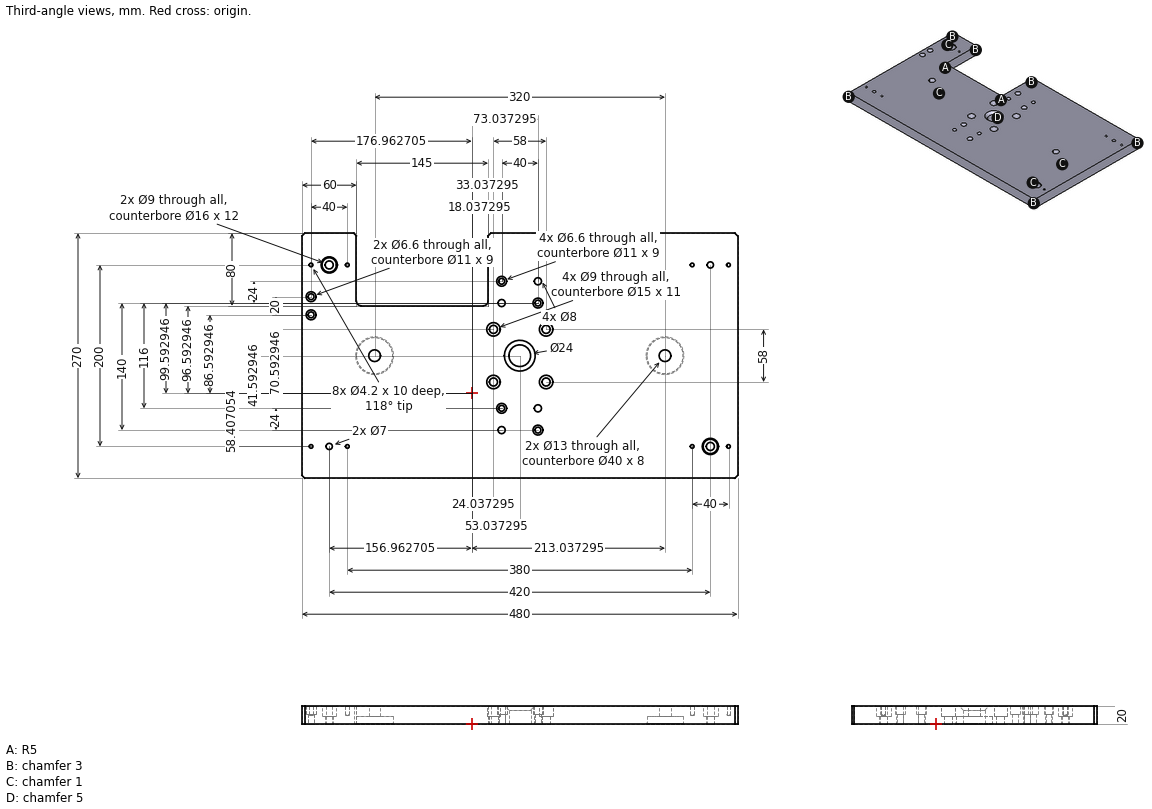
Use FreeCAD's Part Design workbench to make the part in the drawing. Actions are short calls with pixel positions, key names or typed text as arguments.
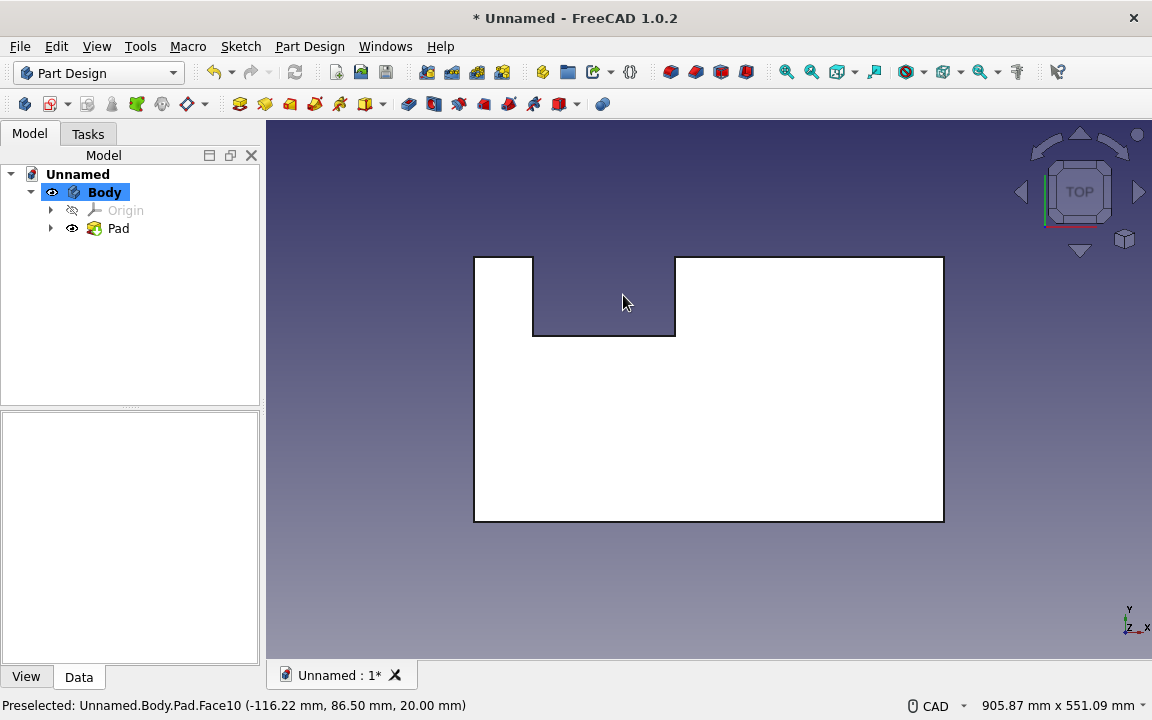
scroll(533, 335, up, 4)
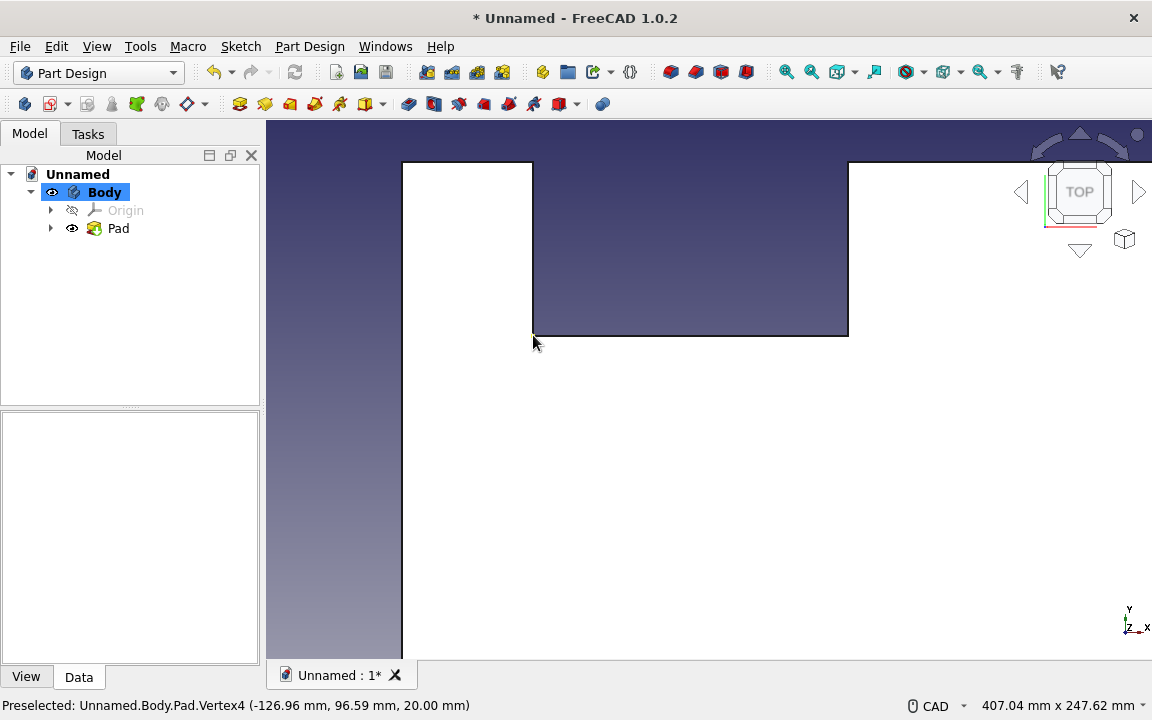
key(v)
key(f)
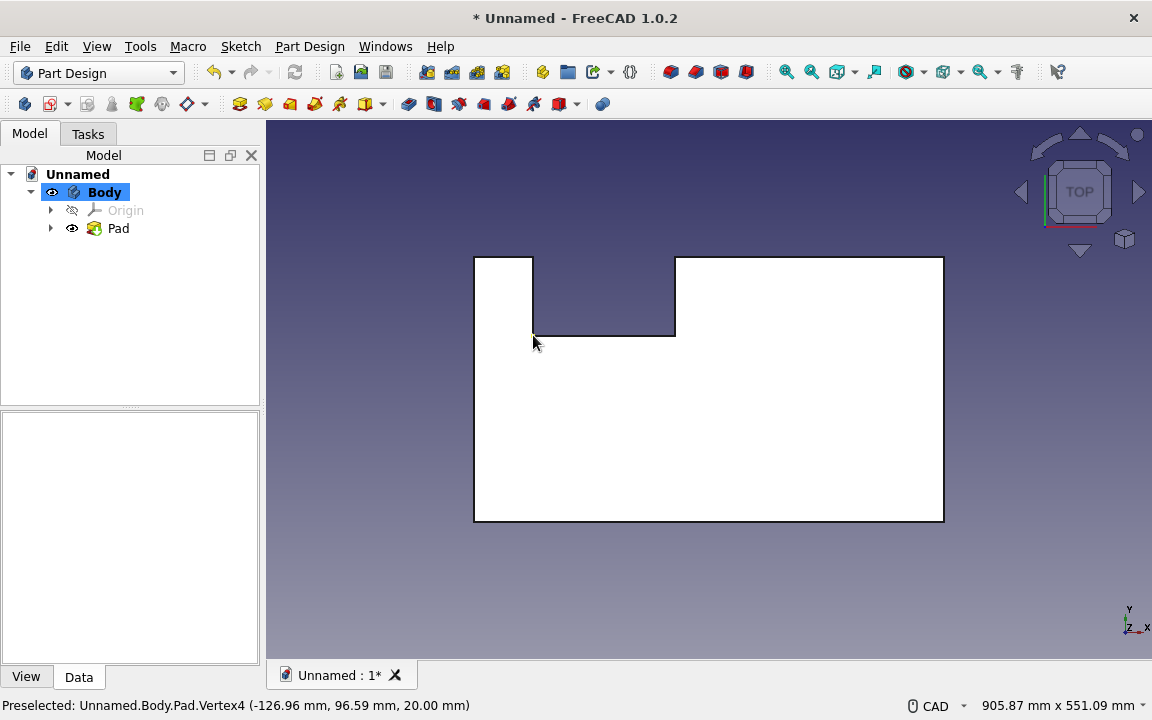
key(1)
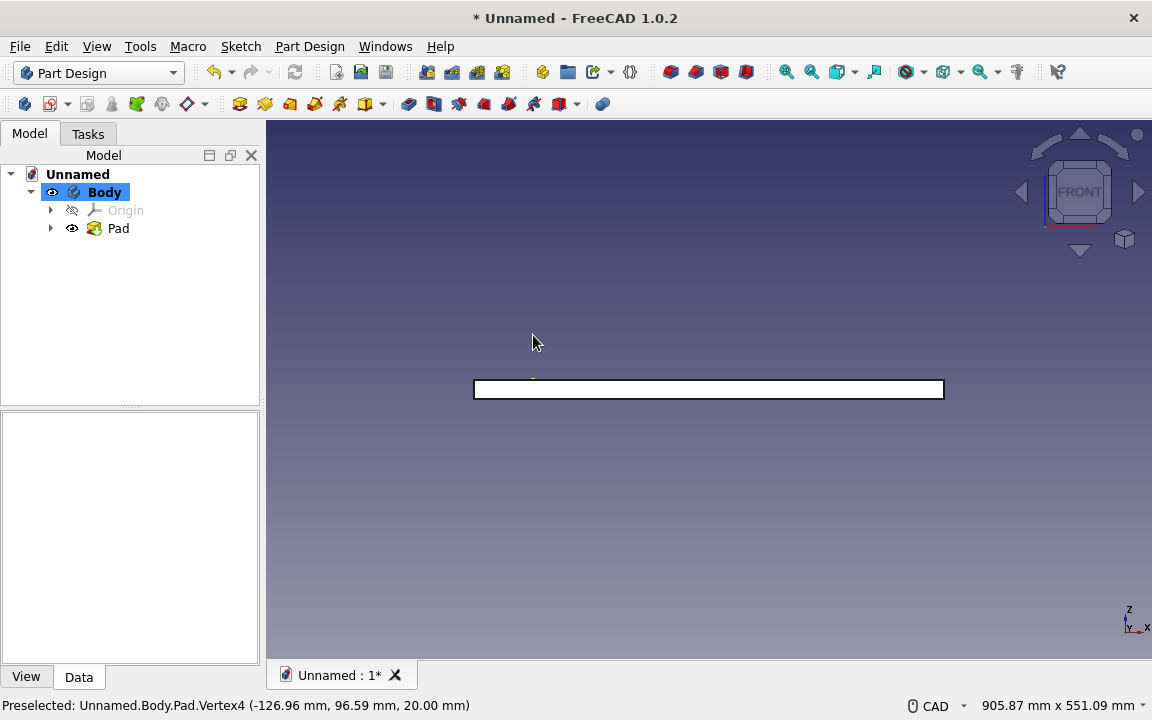
scroll(533, 388, up, 4)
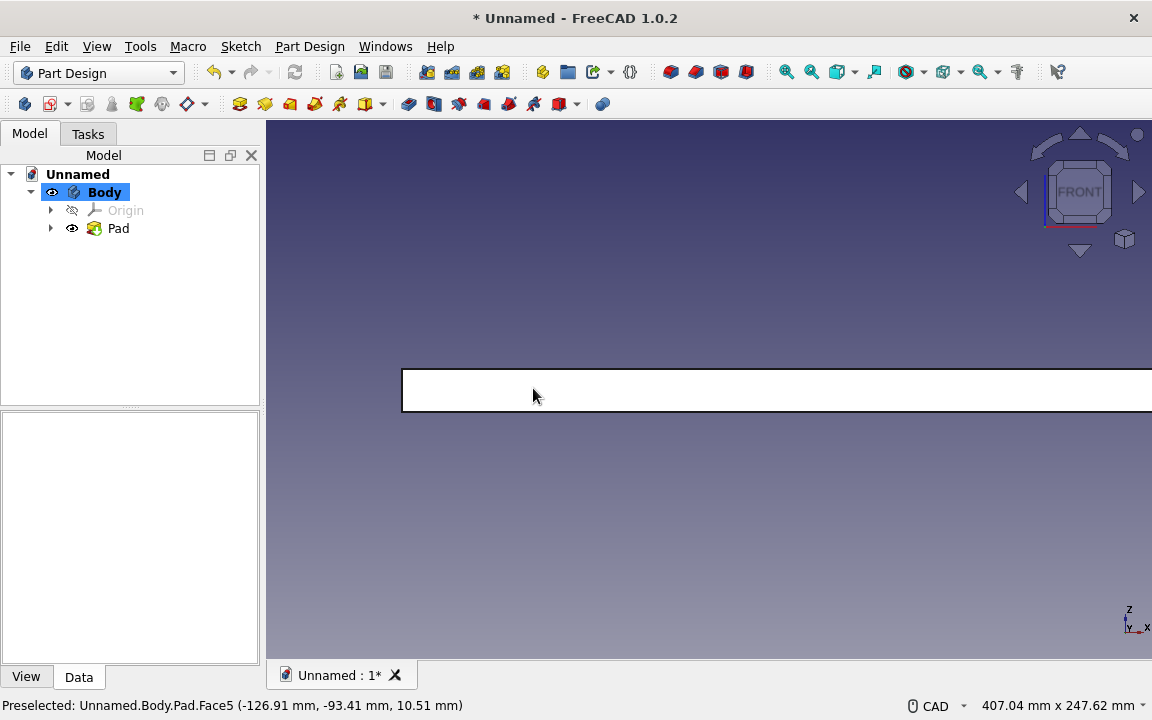
key(v)
key(f)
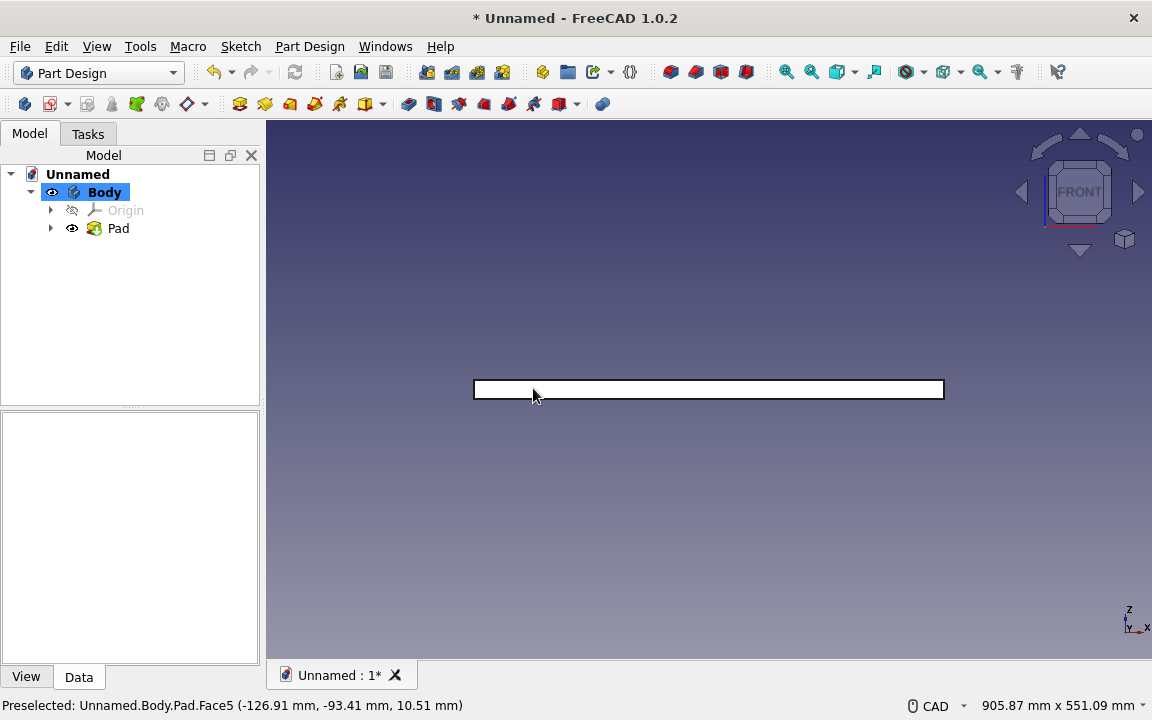
key(3)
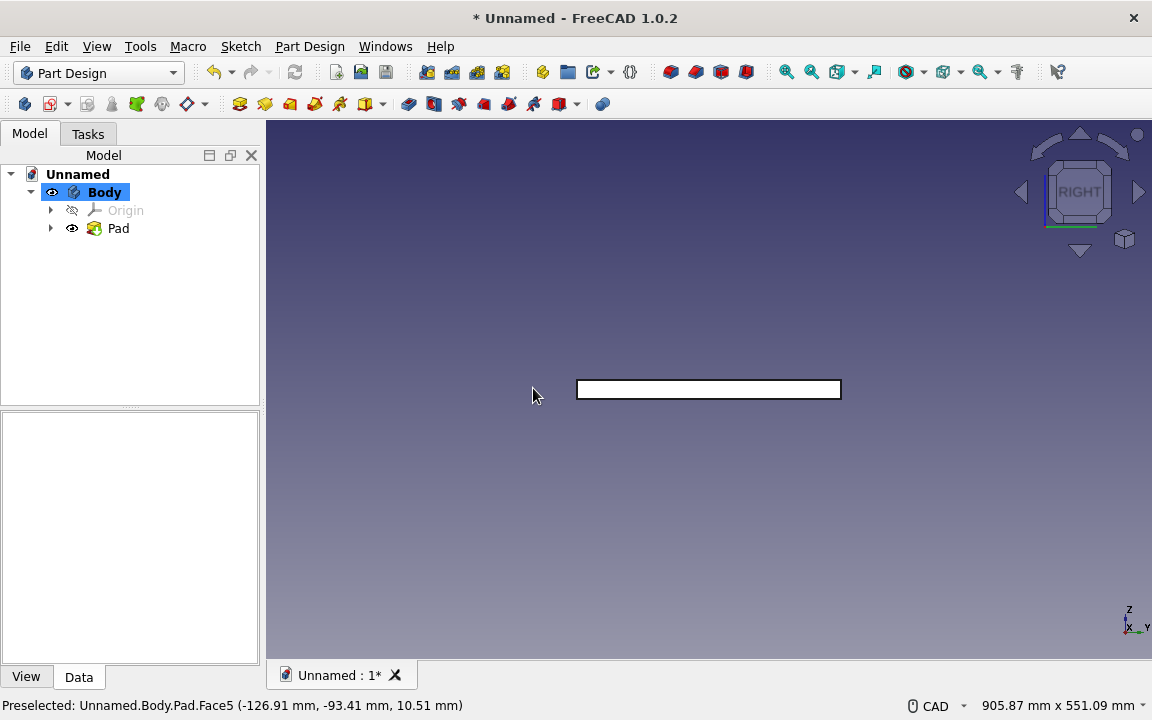
click(787, 72)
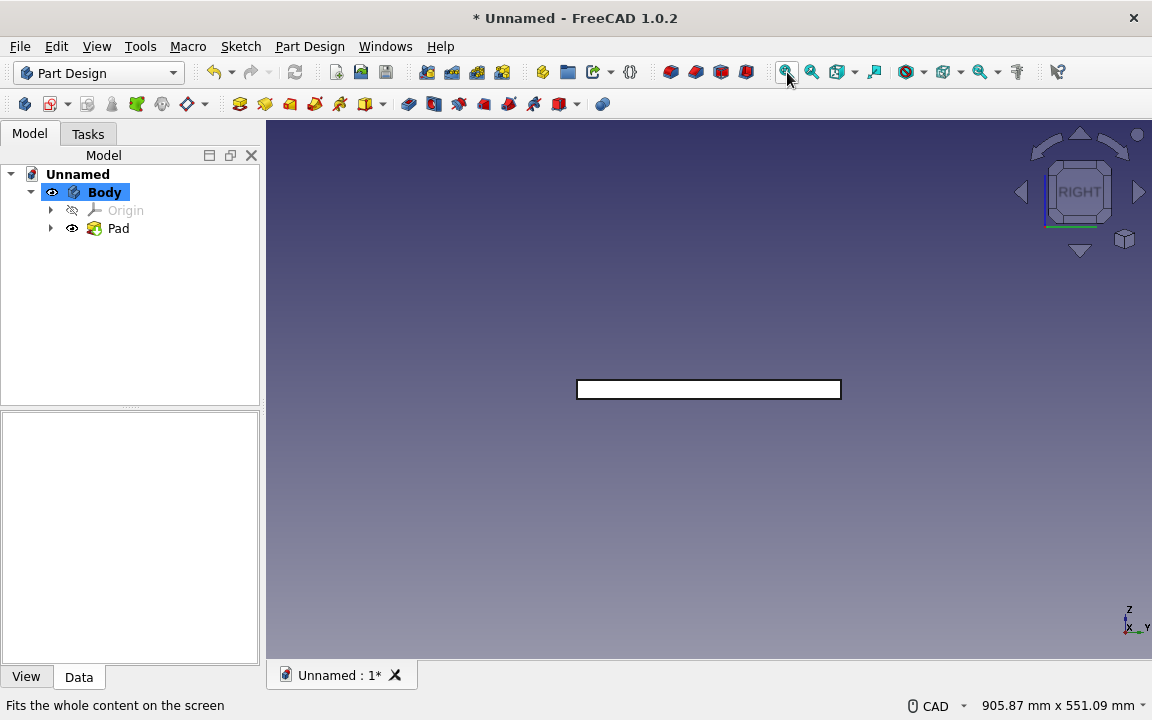
scroll(763, 388, up, 4)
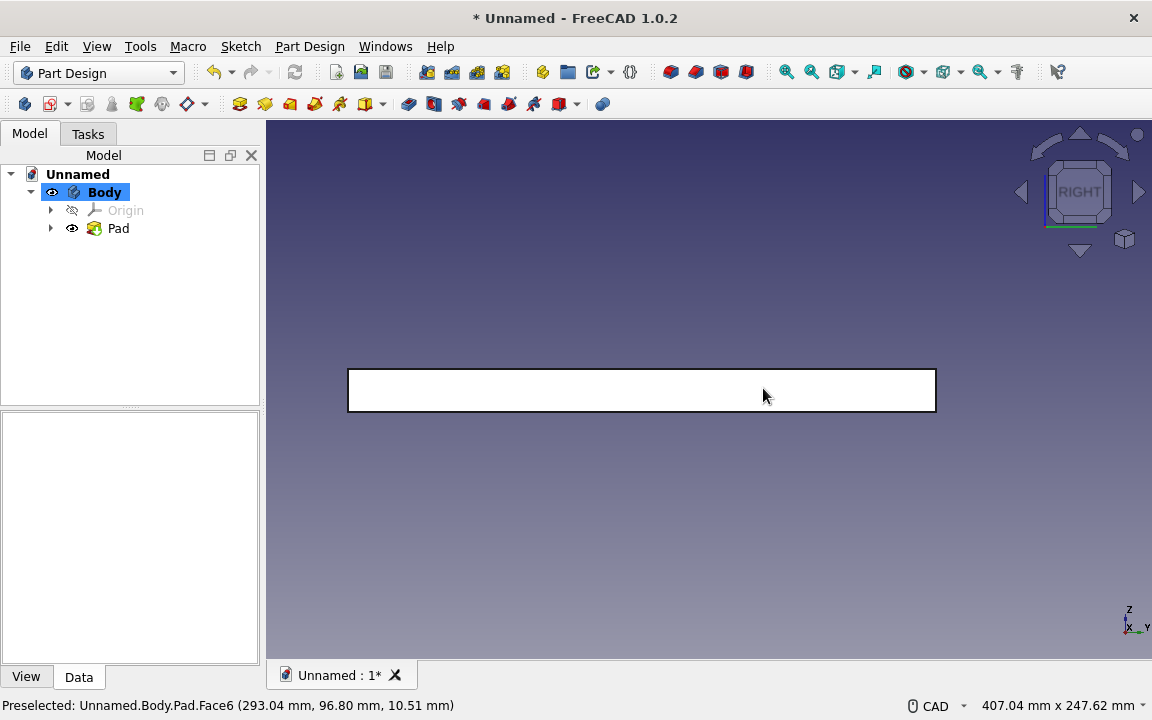
key(v)
key(f)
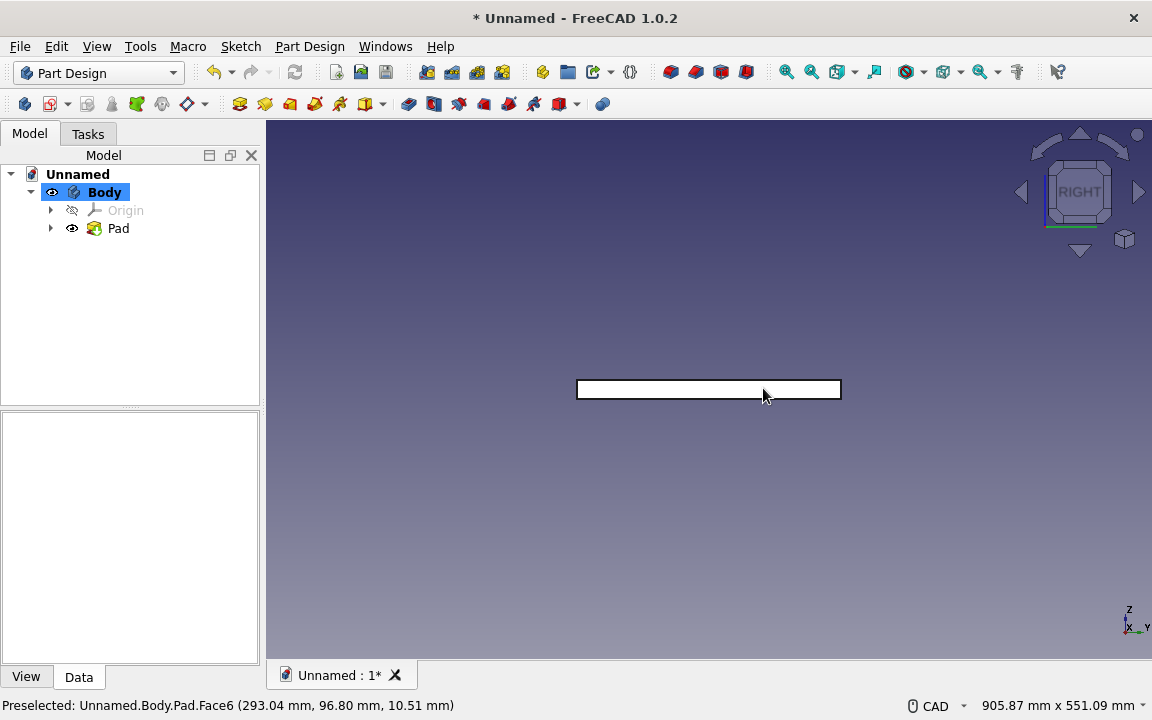
key(5)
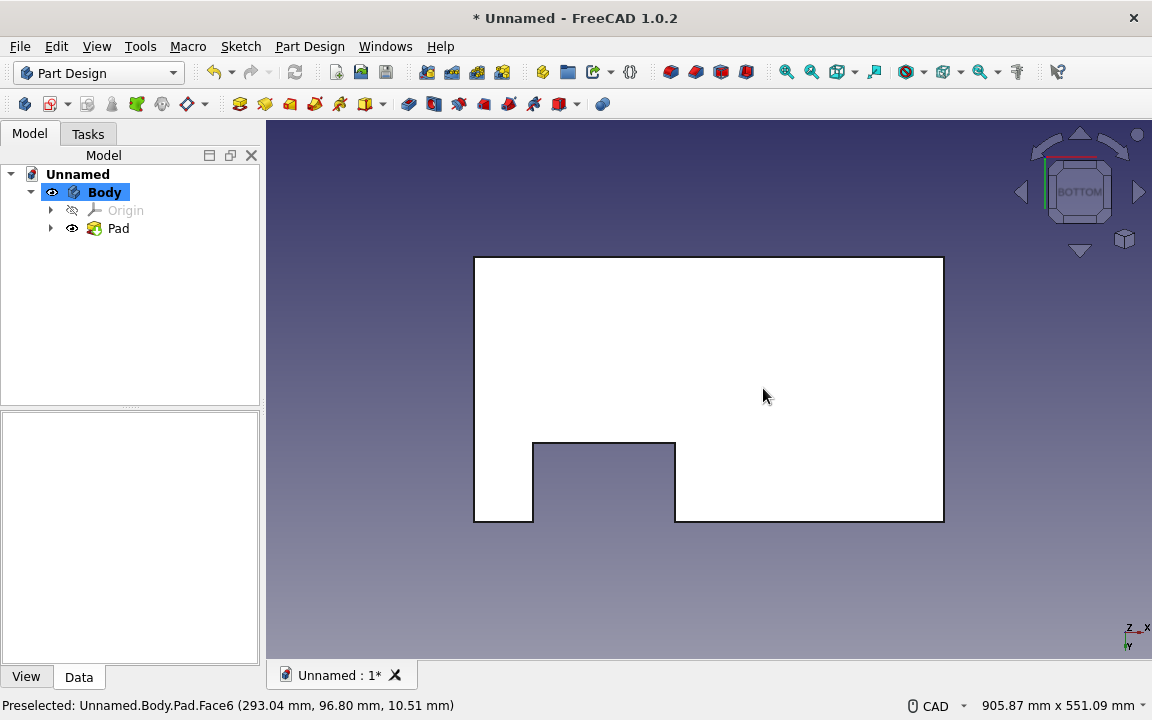
scroll(533, 442, up, 4)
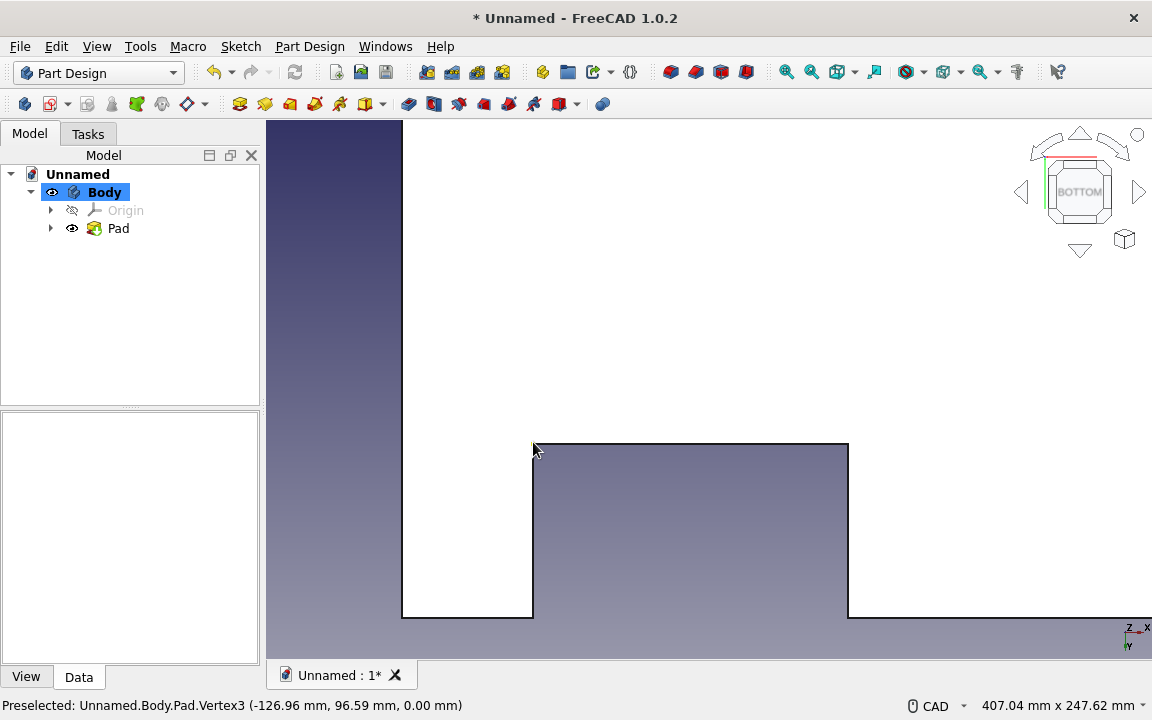
key(v)
key(f)